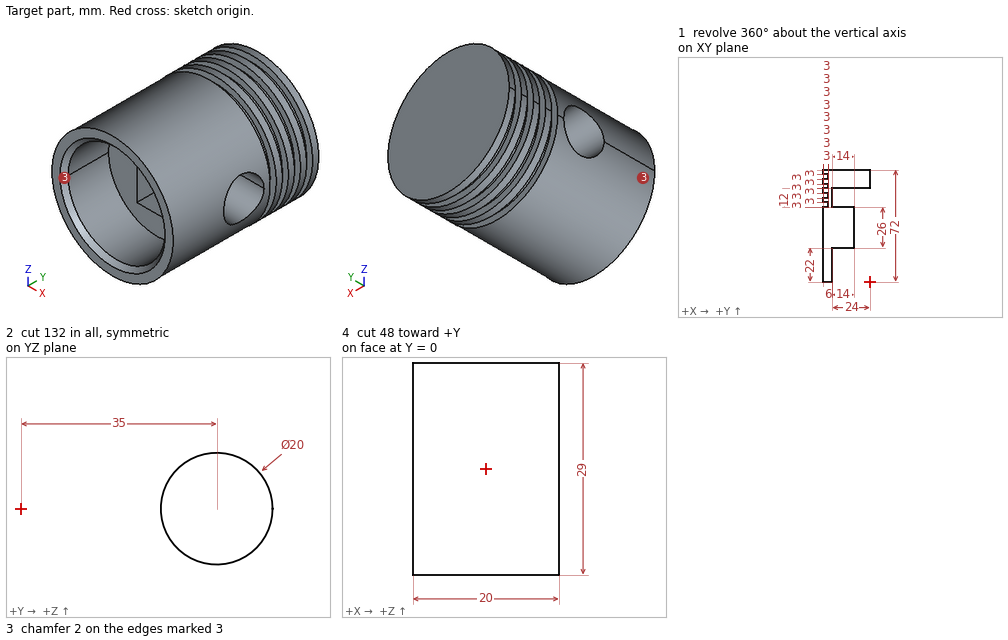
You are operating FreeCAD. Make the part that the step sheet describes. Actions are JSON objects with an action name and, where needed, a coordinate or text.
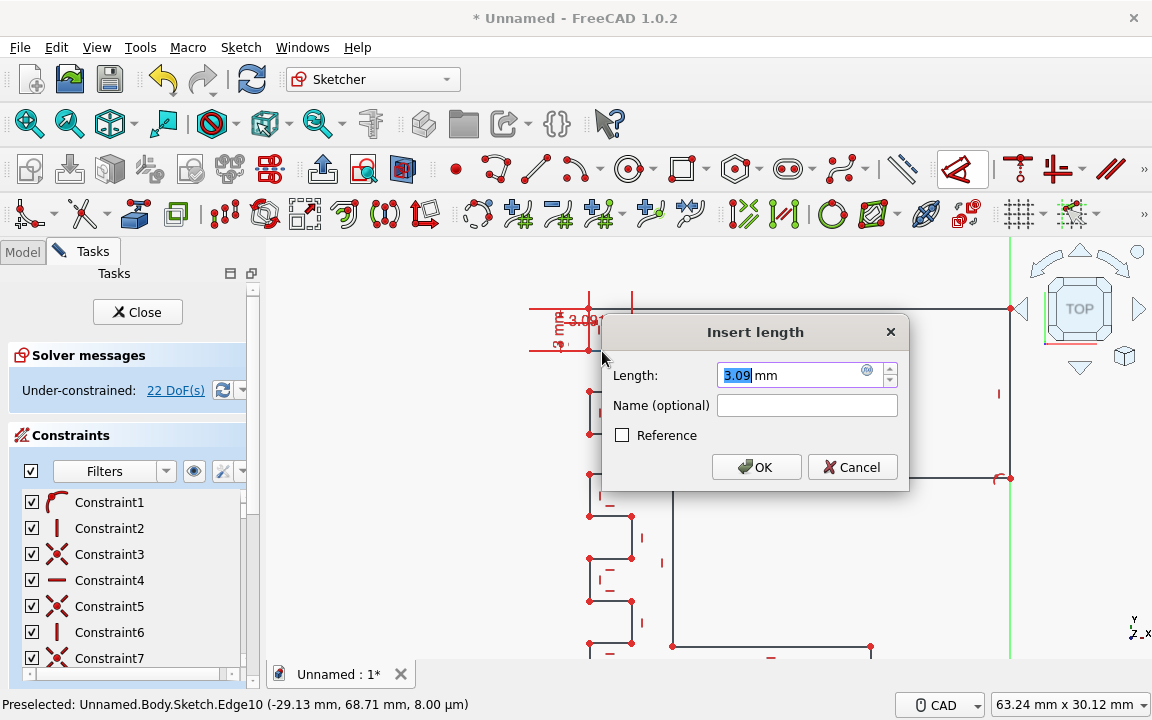
{"action": "type", "text": "3"}
{"action": "key", "text": "Return"}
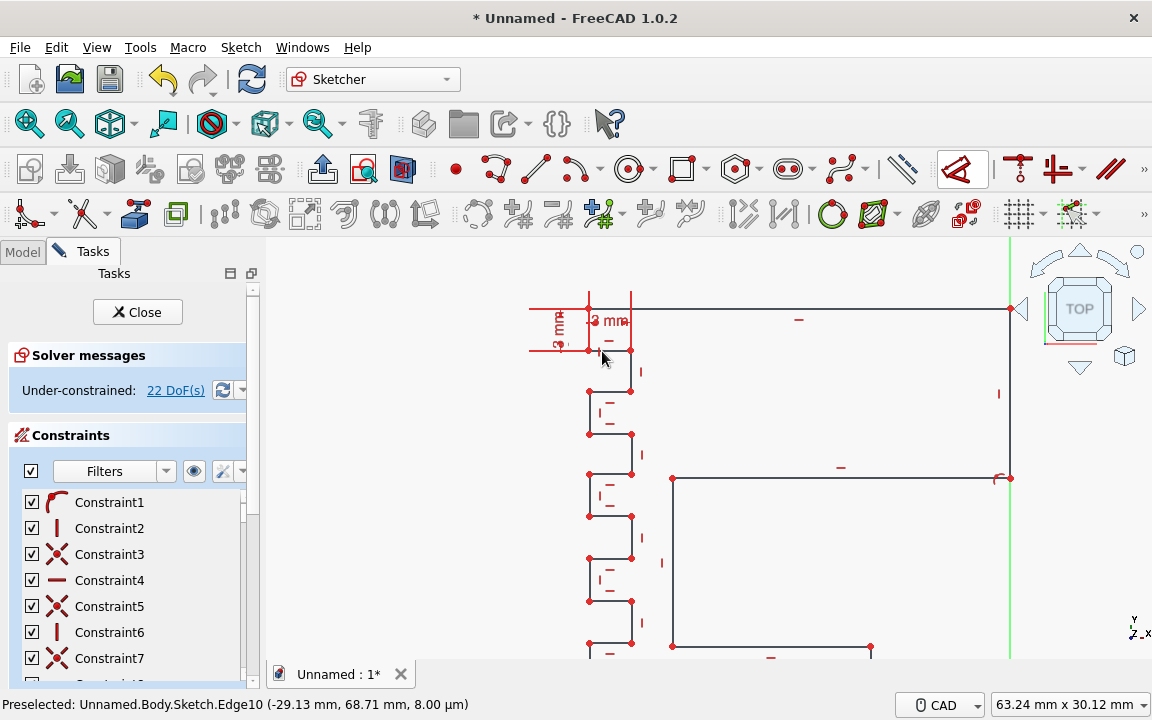
{"action": "left_click", "coordinate": [631, 363]}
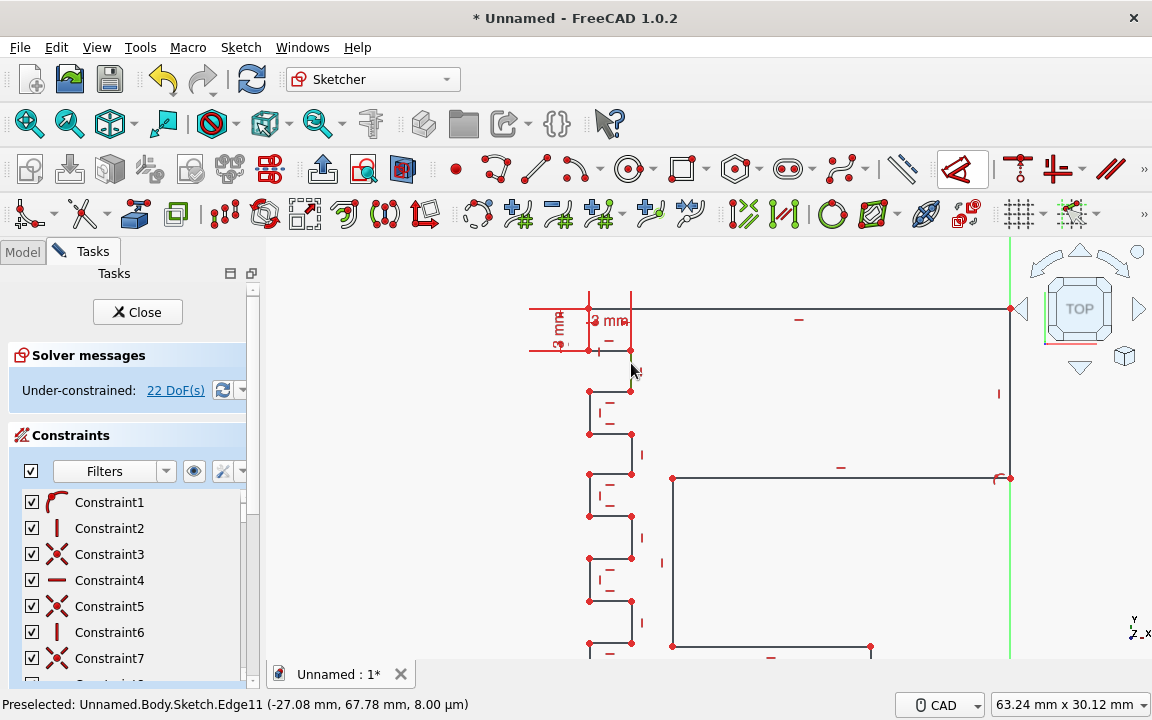
{"action": "left_click", "coordinate": [982, 170]}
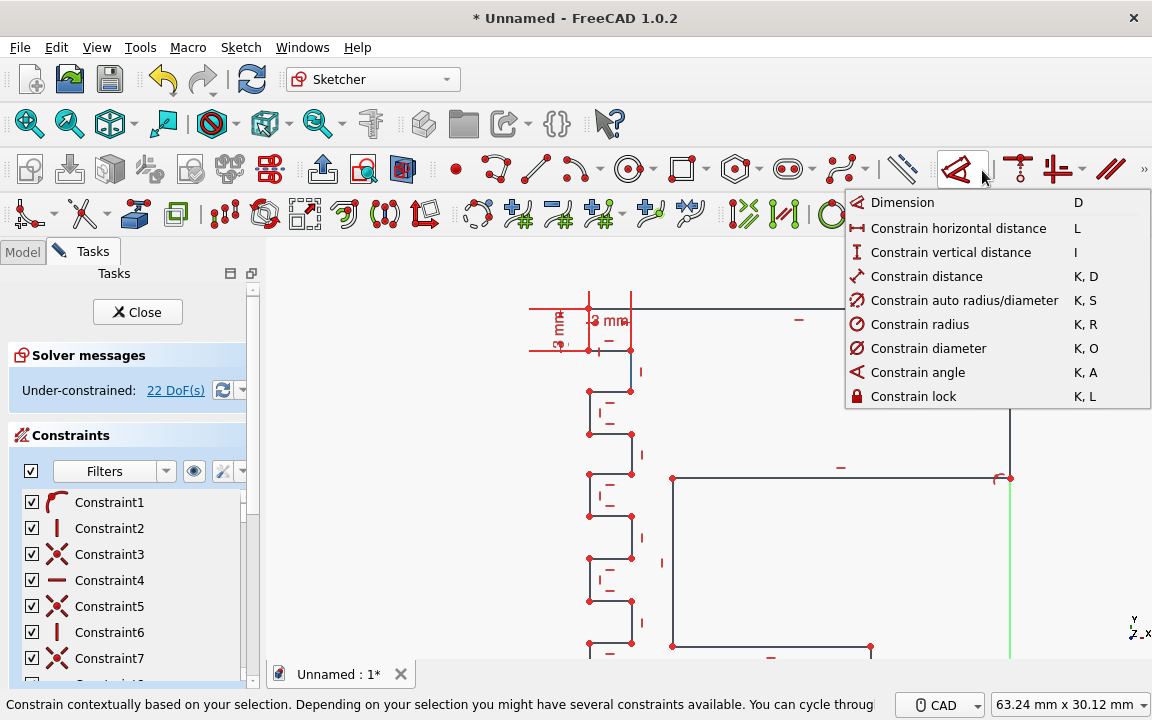
{"action": "left_click", "coordinate": [998, 252]}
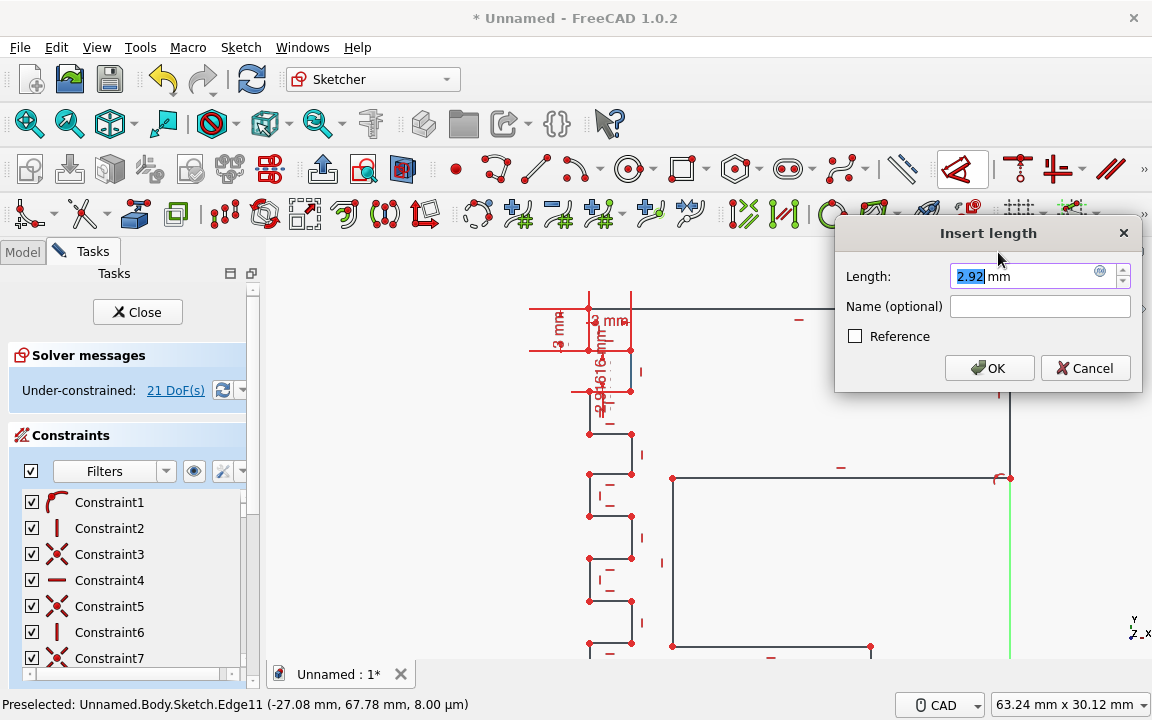
{"action": "type", "text": "3"}
{"action": "key", "text": "Return"}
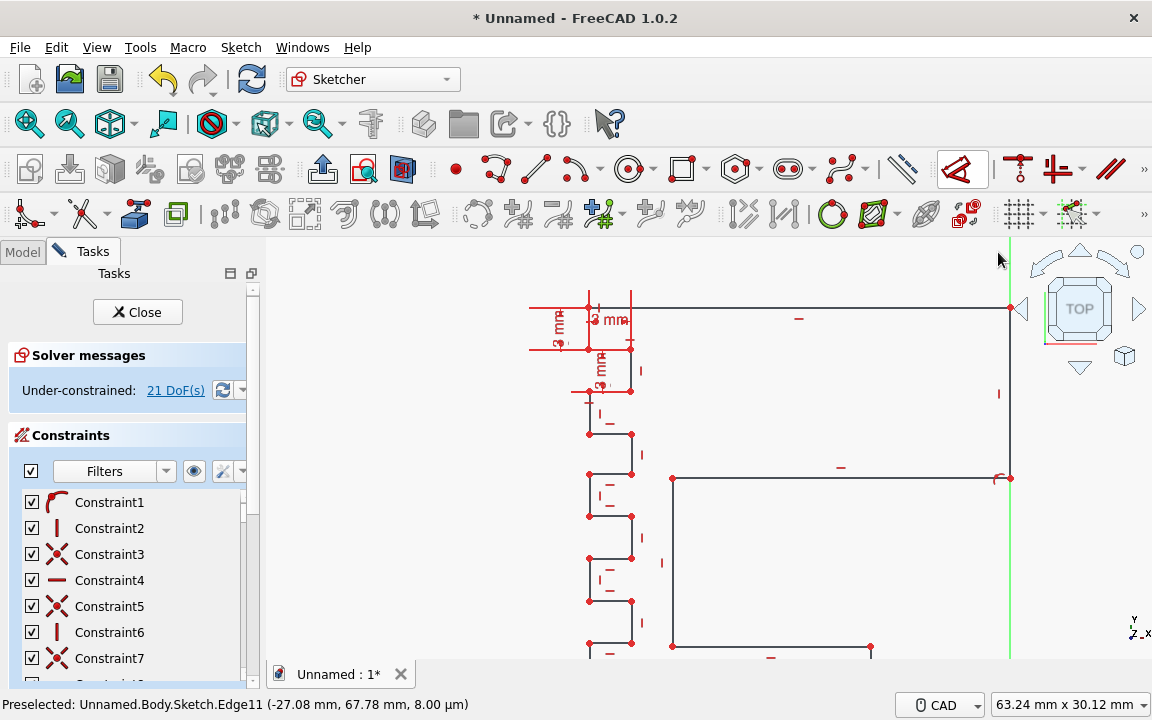
{"action": "left_click", "coordinate": [618, 392]}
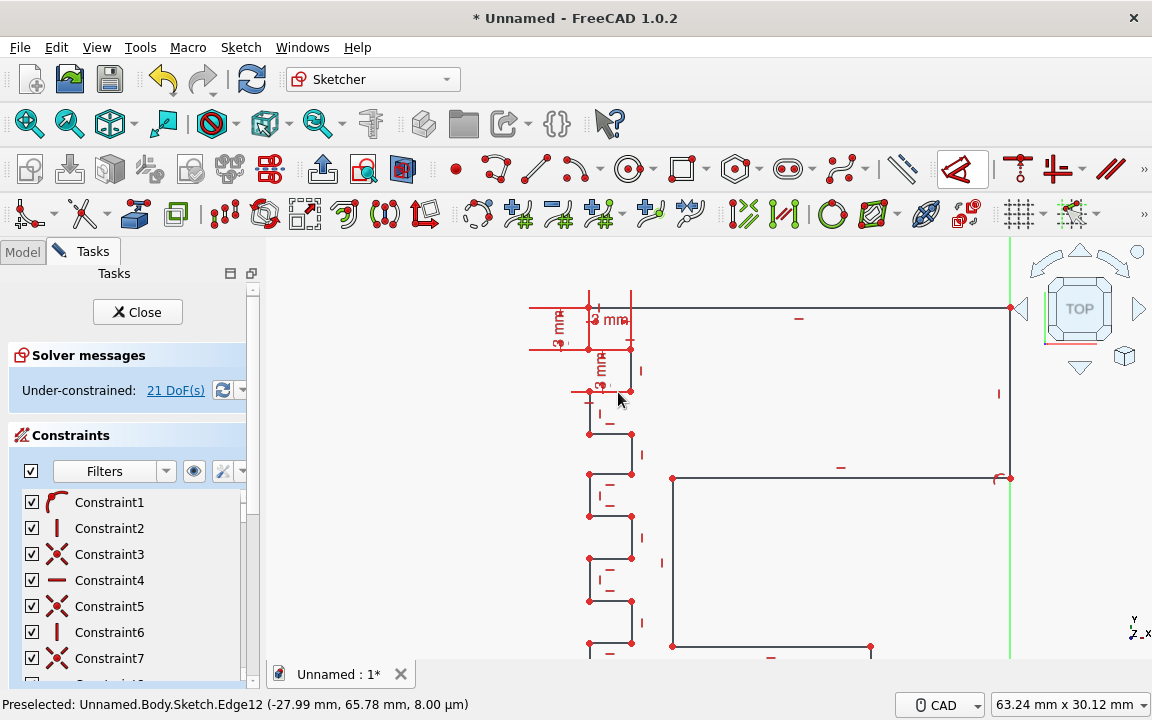
{"action": "key", "text": "l"}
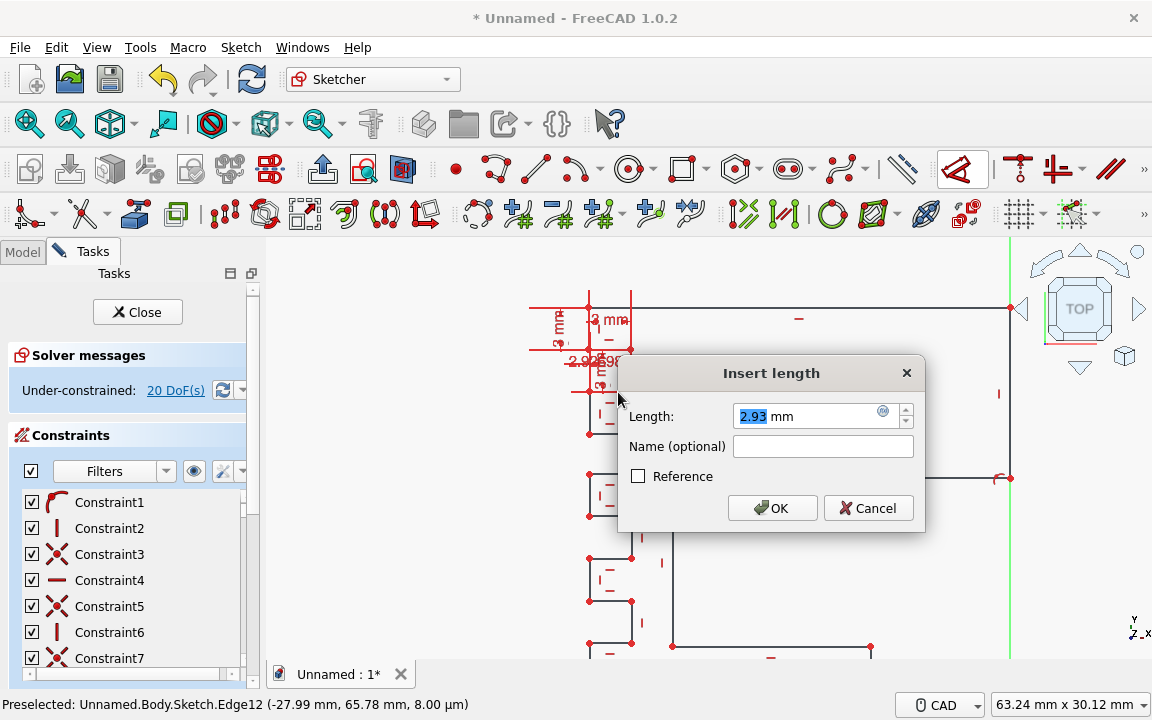
{"action": "type", "text": "3"}
{"action": "key", "text": "Return"}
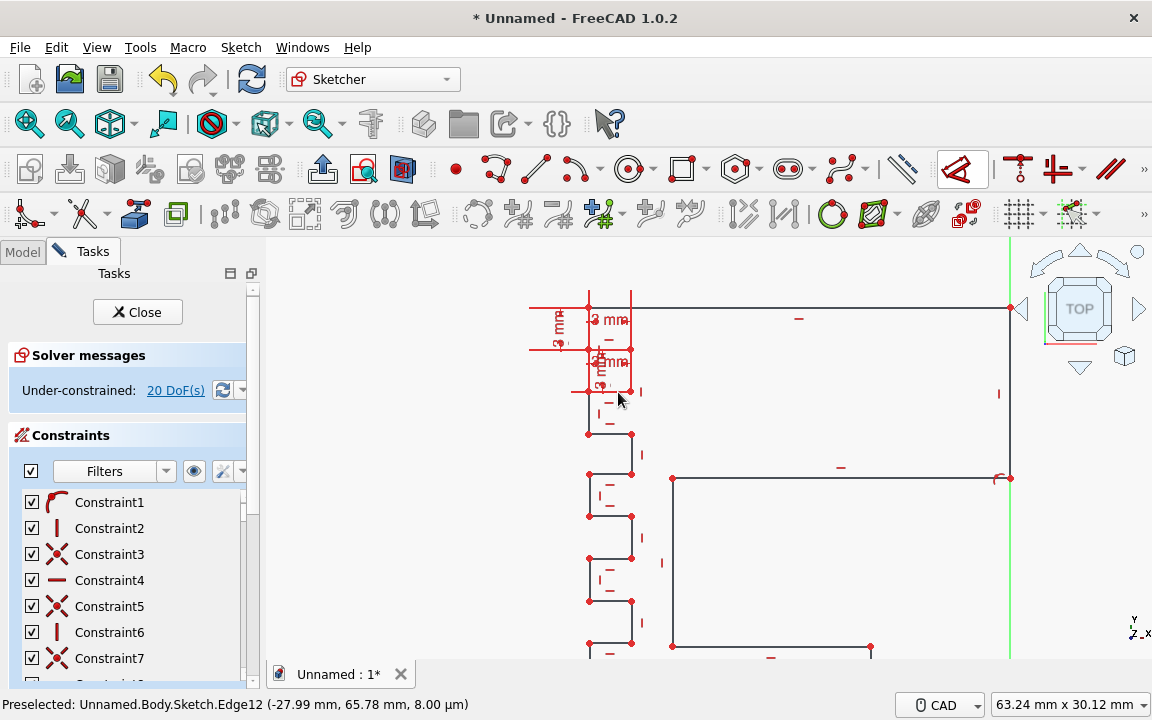
{"action": "left_click", "coordinate": [589, 405]}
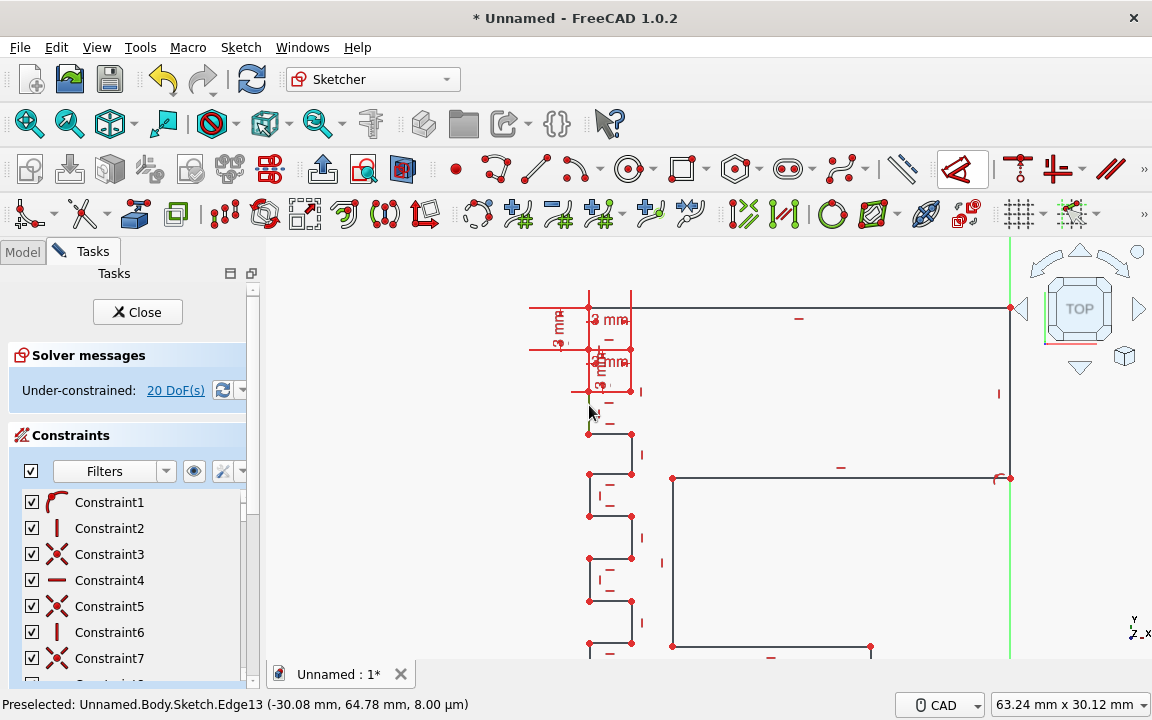
{"action": "left_click", "coordinate": [982, 170]}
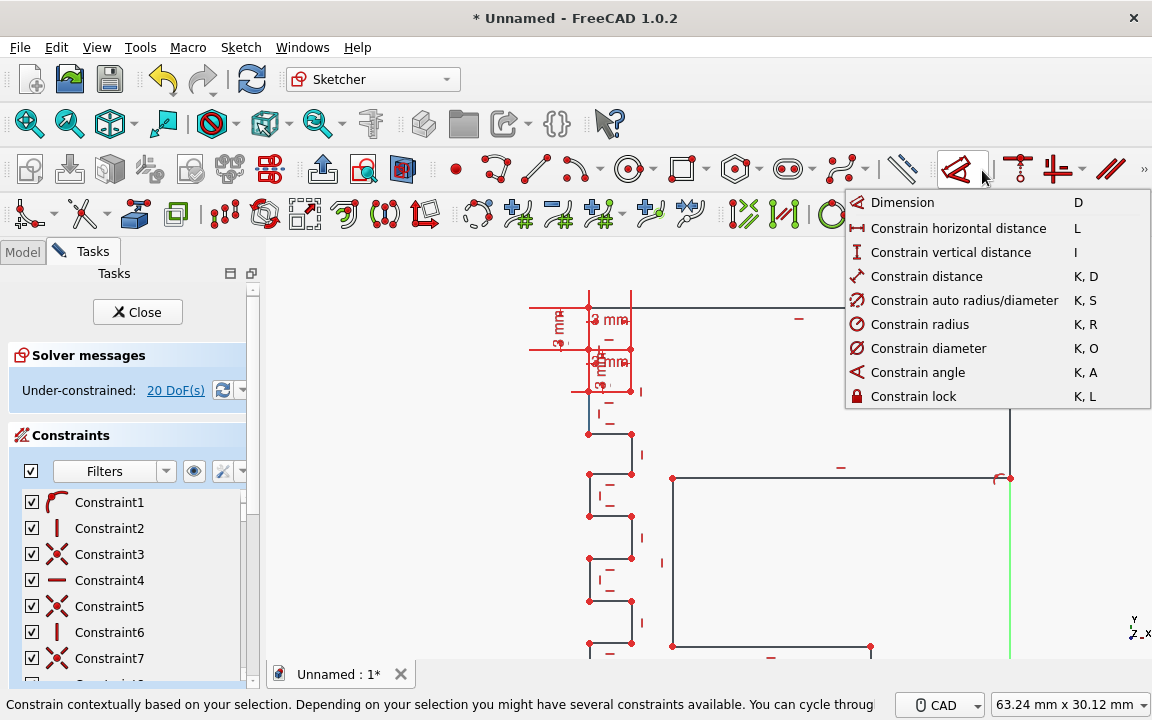
{"action": "left_click", "coordinate": [998, 252]}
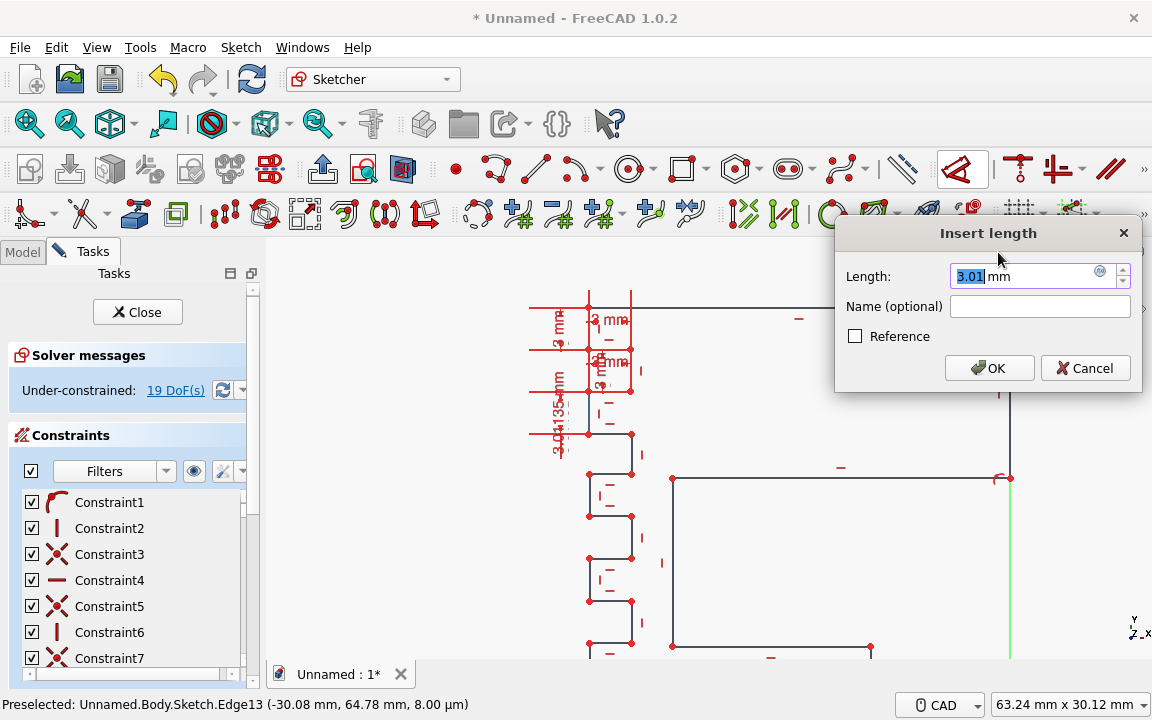
{"action": "type", "text": "3"}
{"action": "key", "text": "Return"}